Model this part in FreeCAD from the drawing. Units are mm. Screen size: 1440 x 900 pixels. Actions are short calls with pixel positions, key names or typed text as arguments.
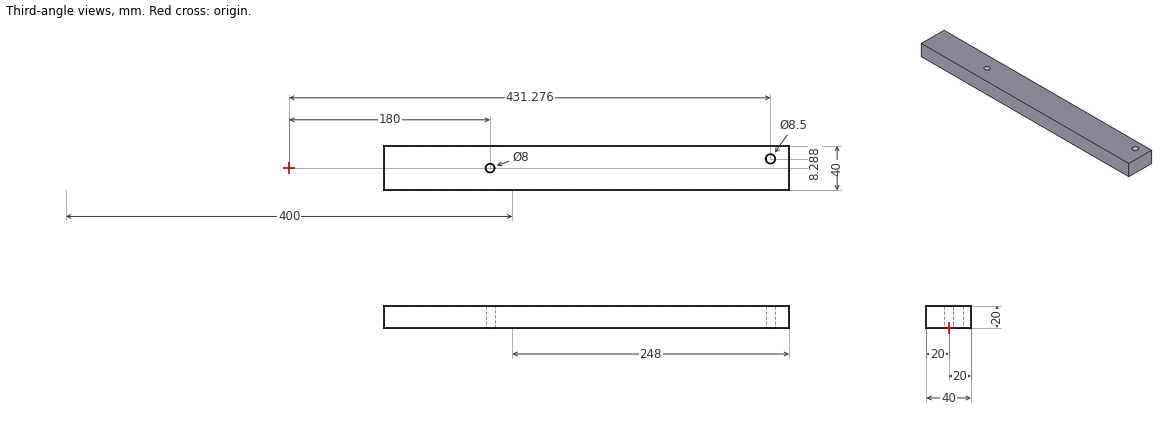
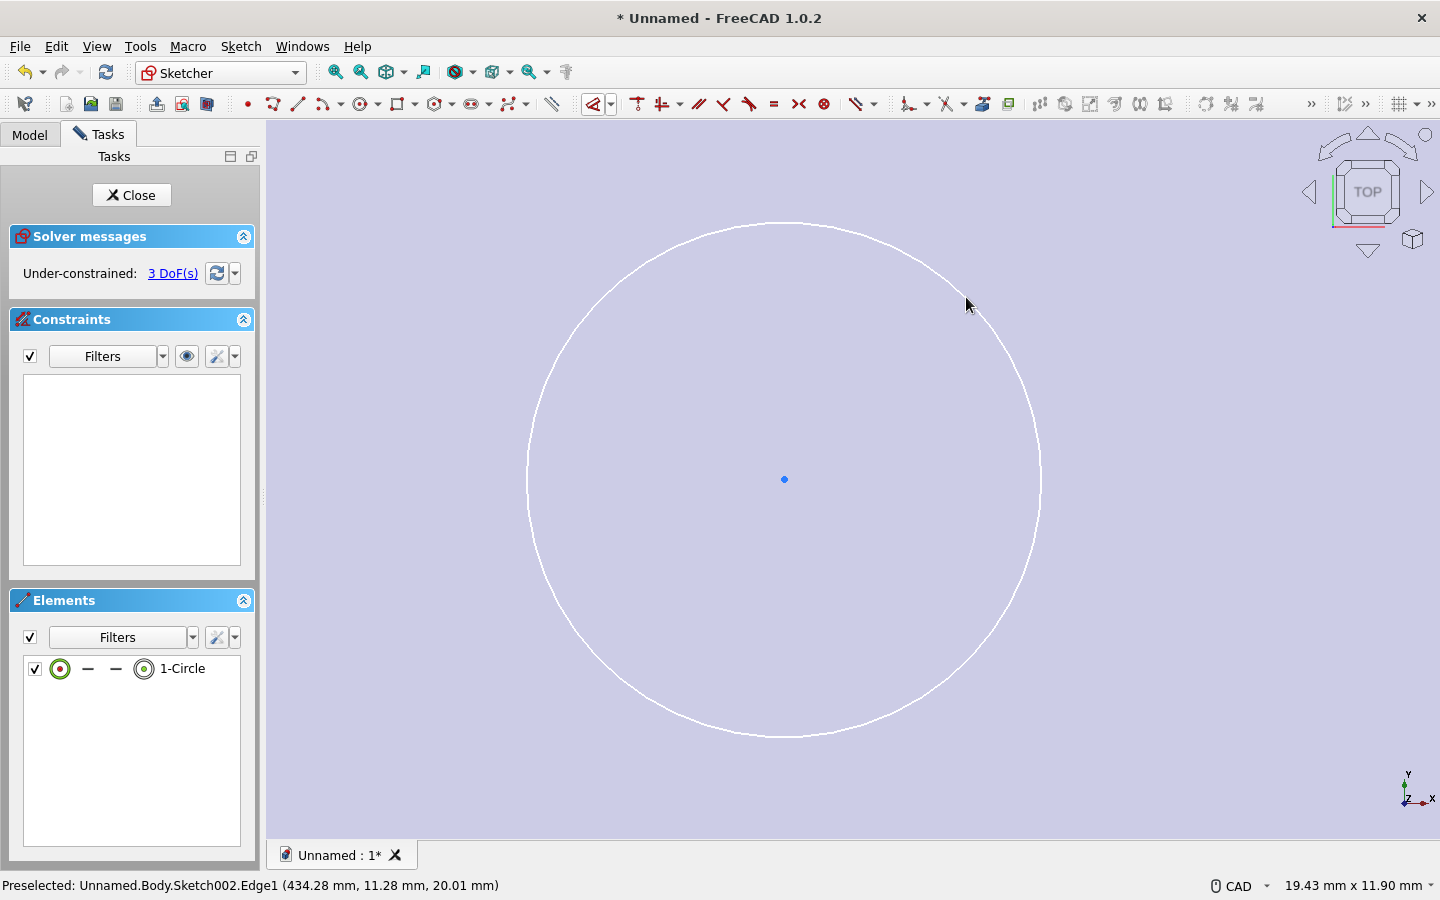
click(965, 297)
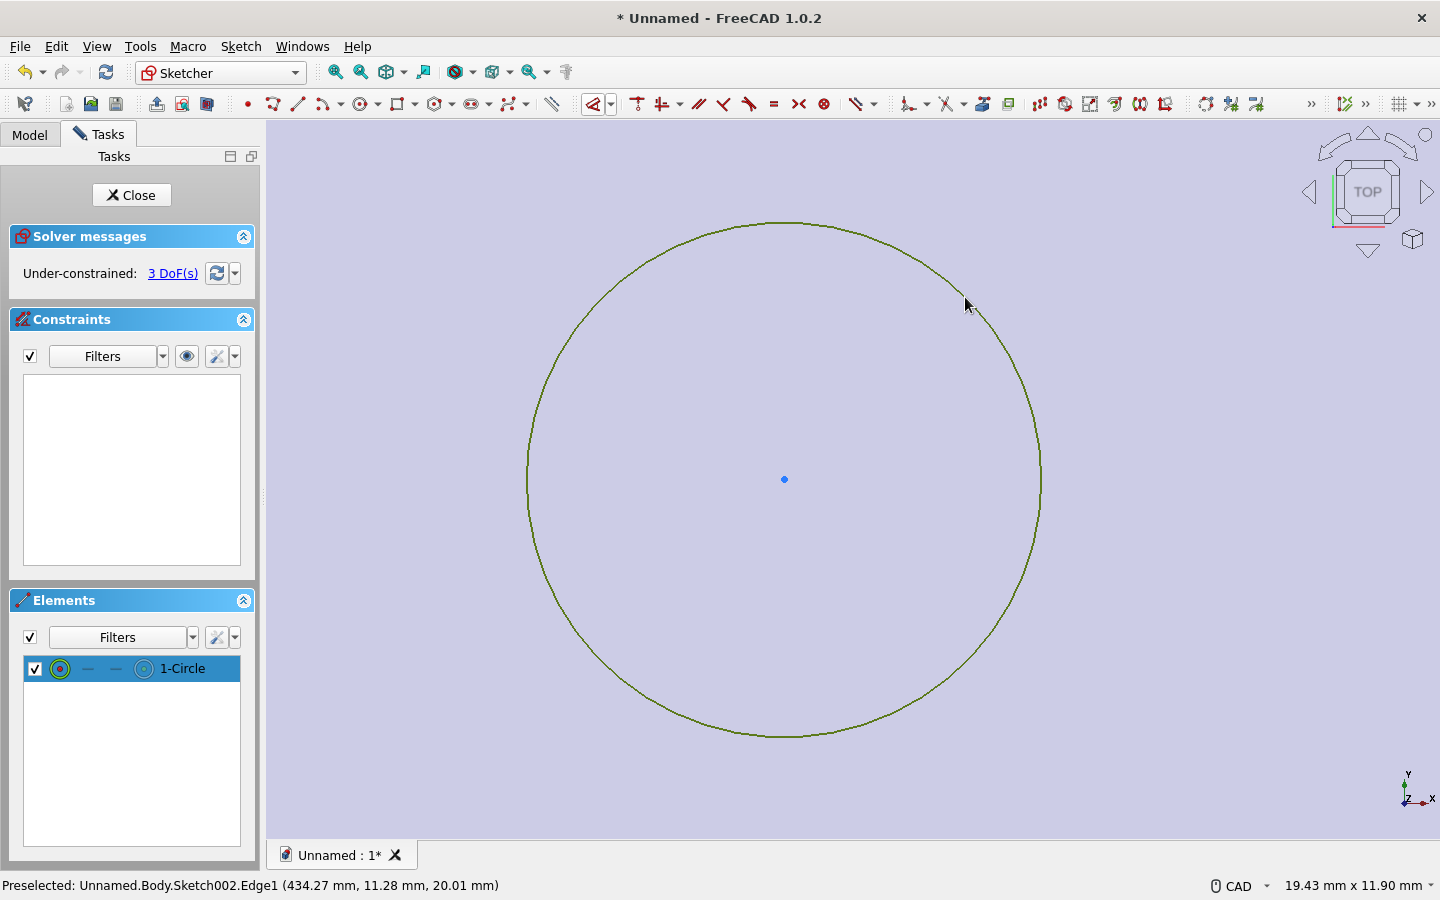
click(610, 104)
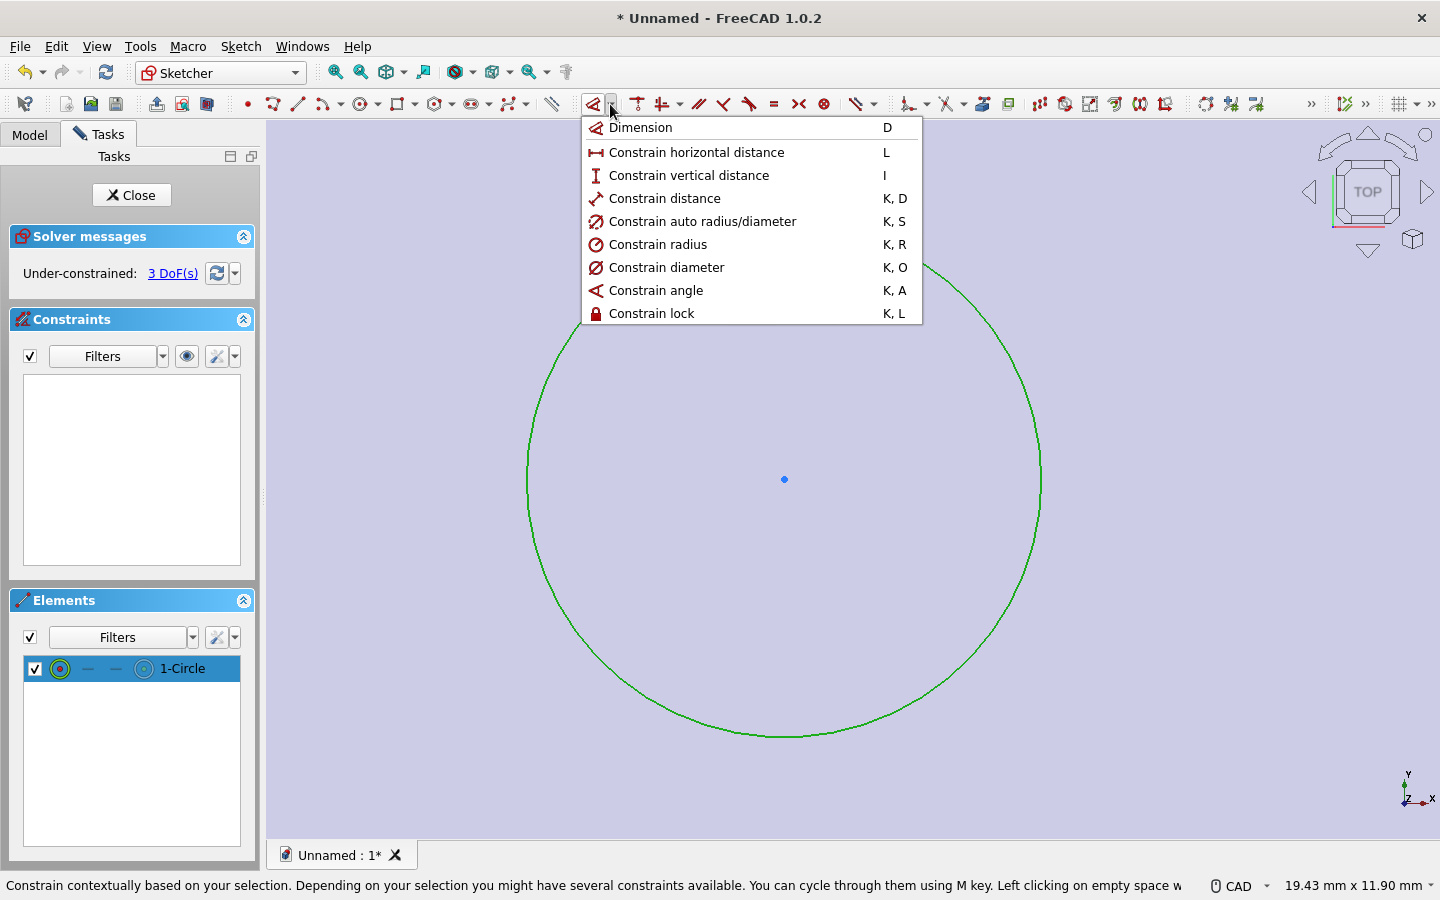
click(752, 268)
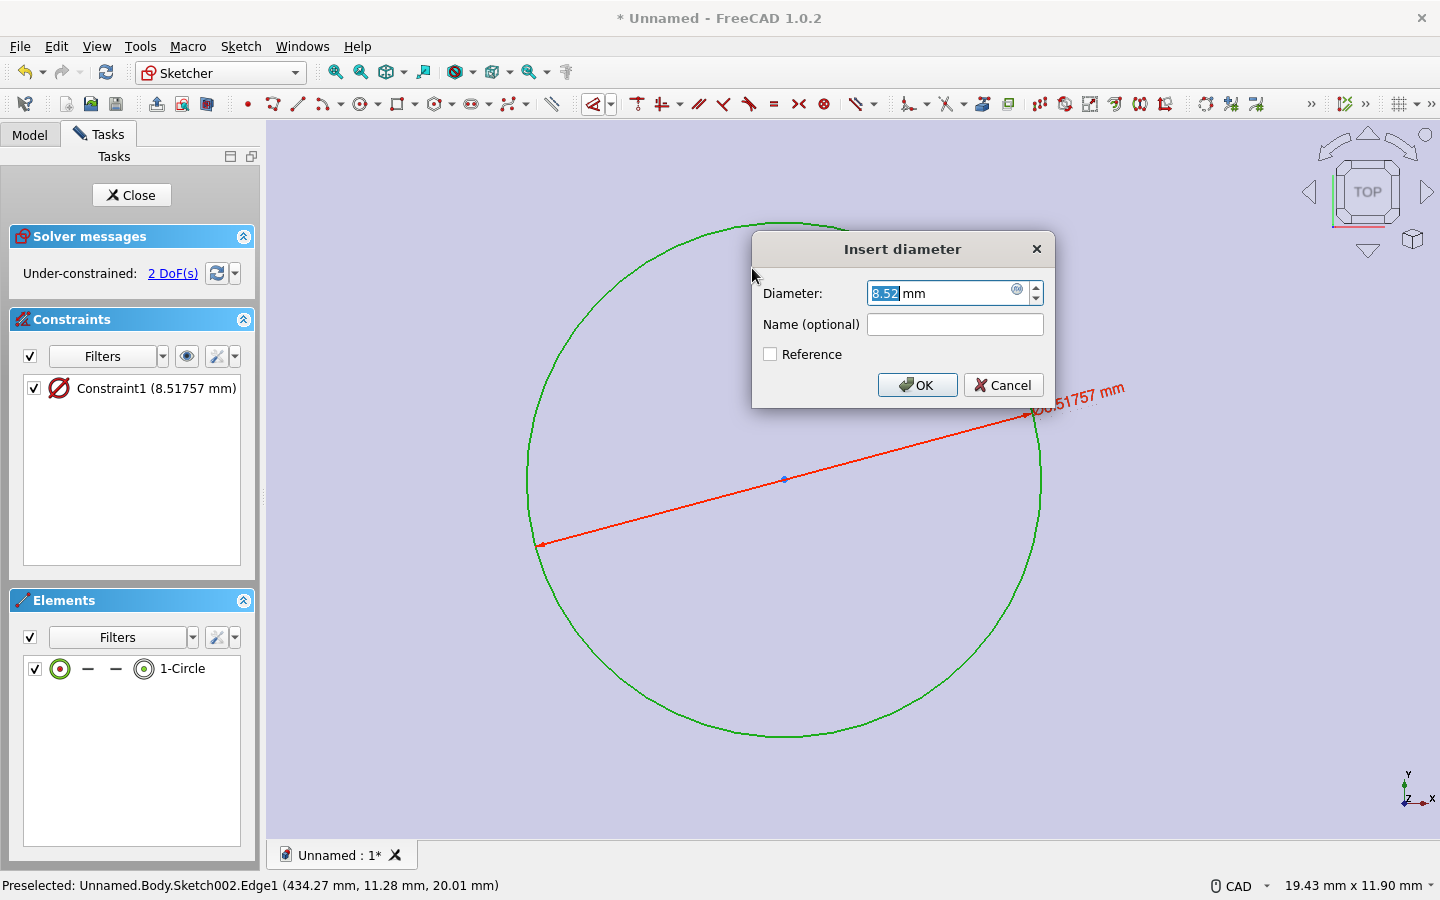
text(8.5)
key(Return)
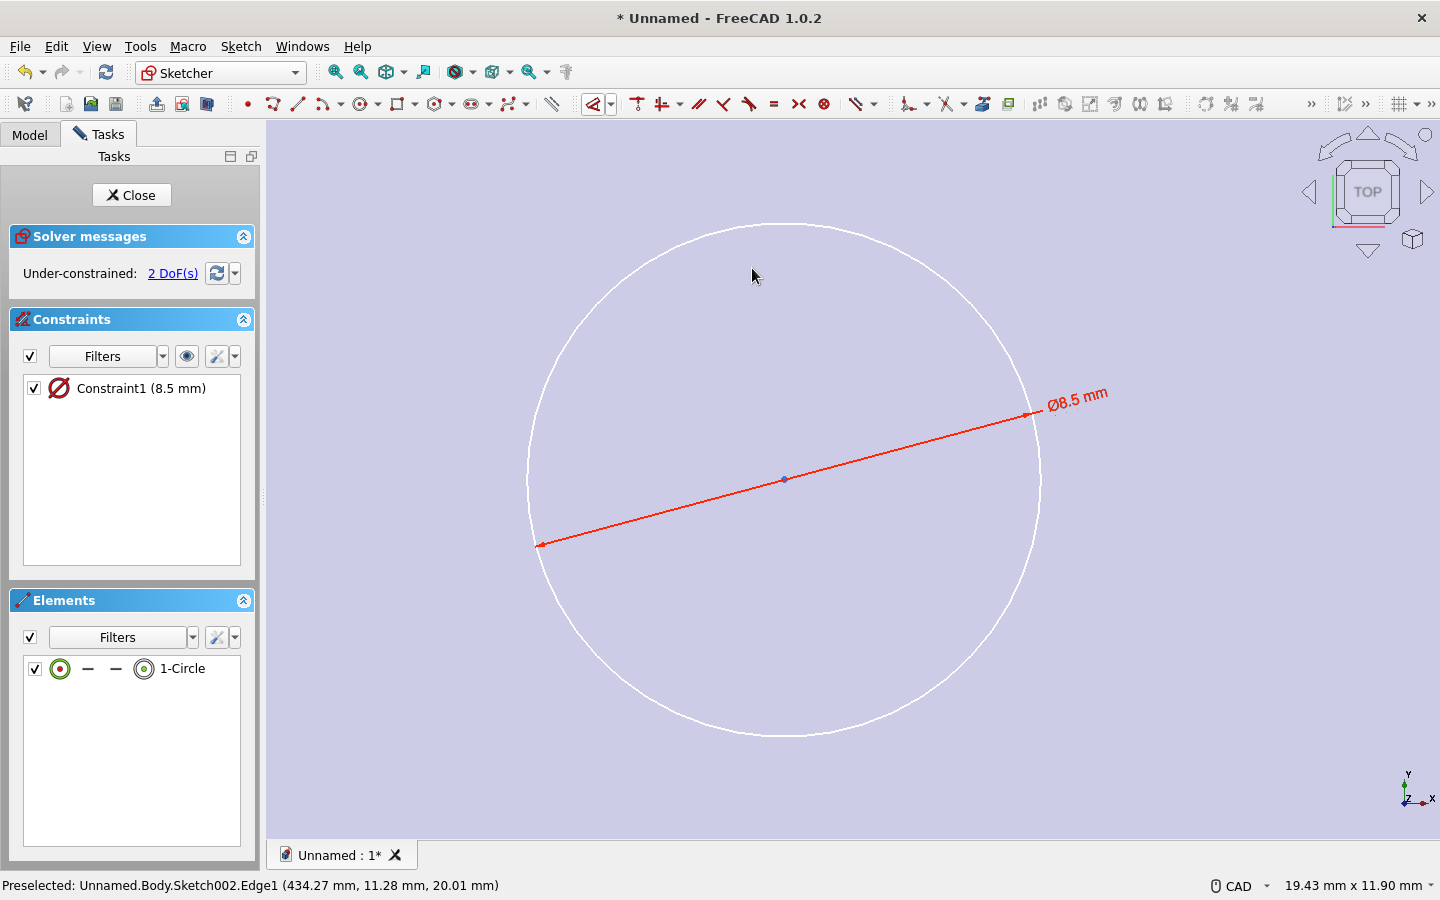
click(784, 480)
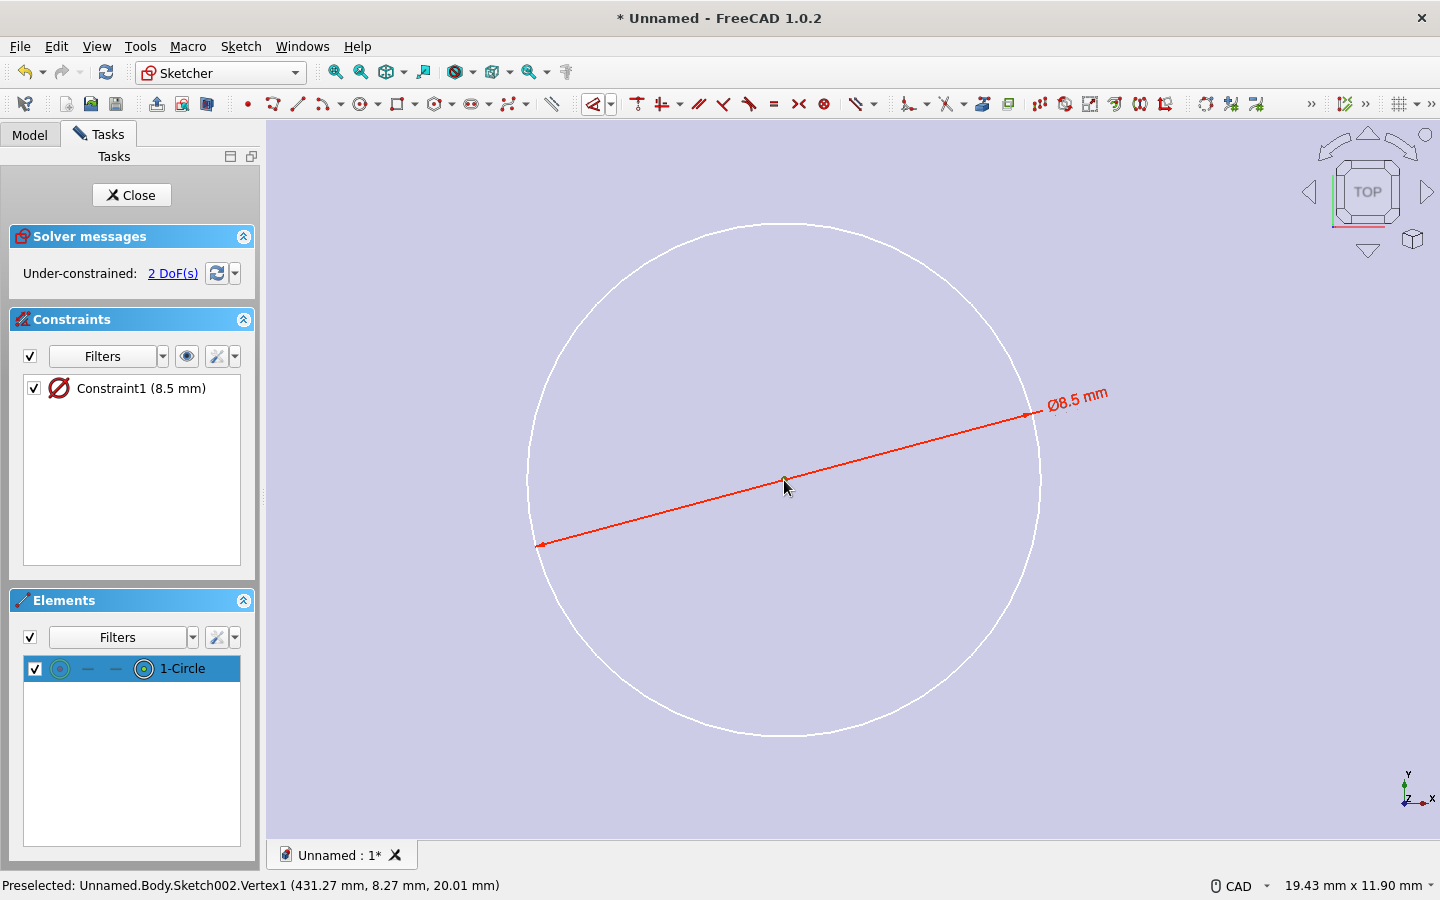
key(i)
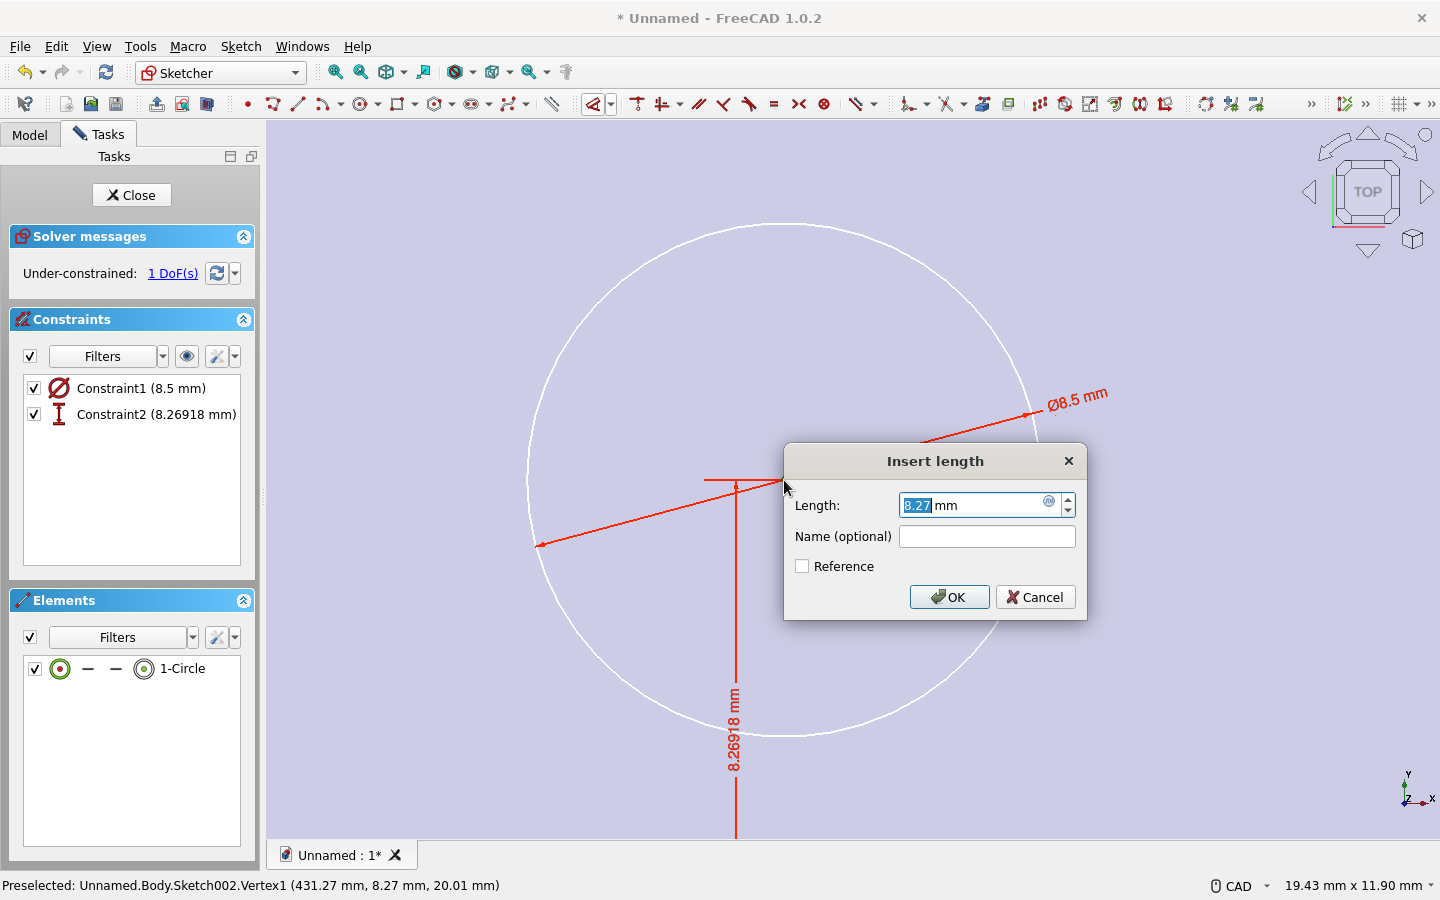
text(8.288)
key(Return)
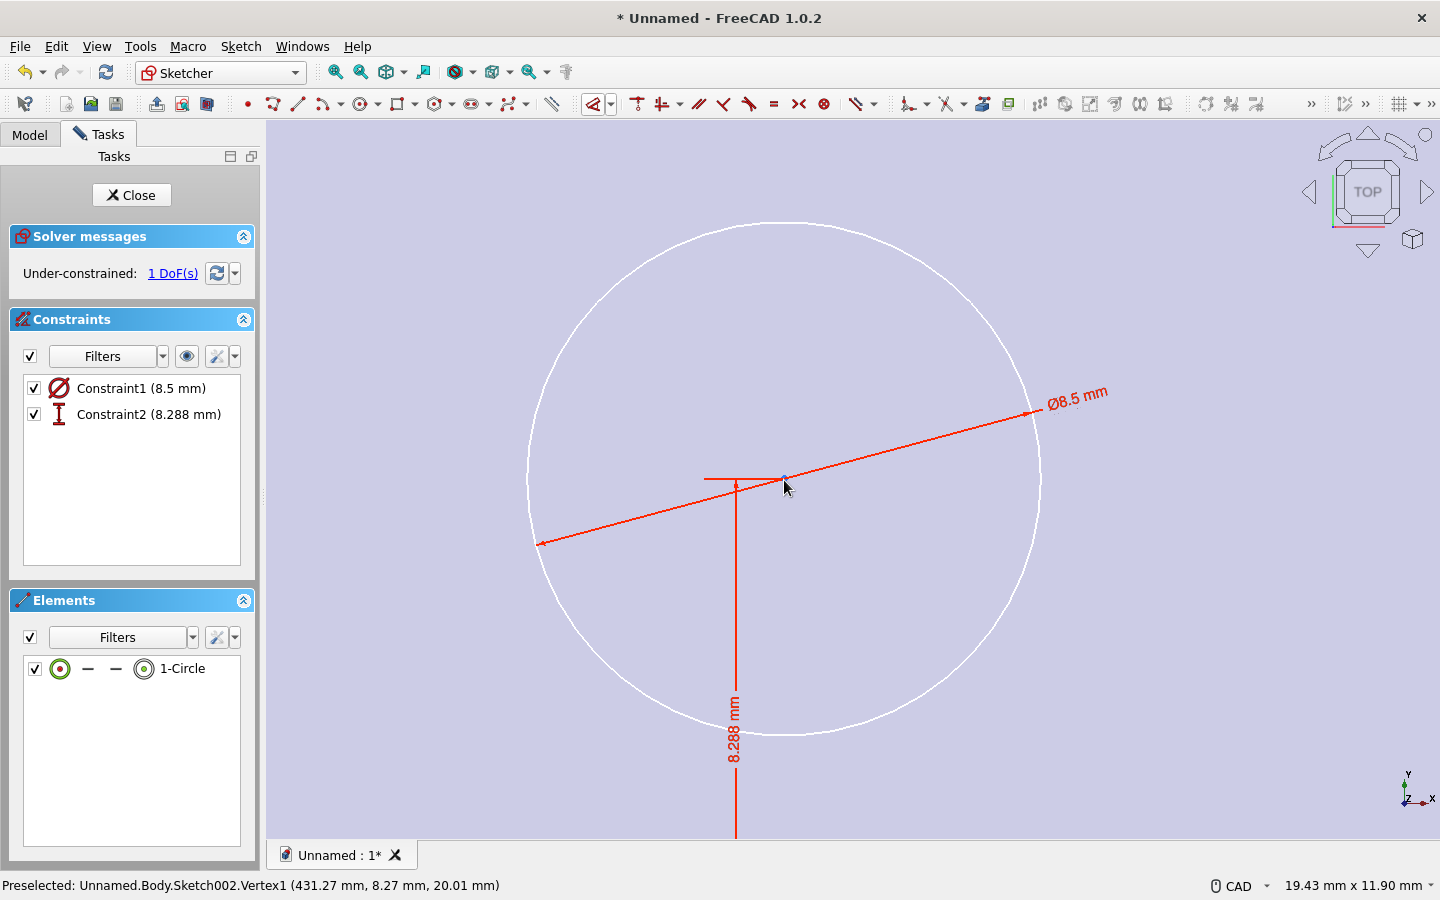
click(784, 479)